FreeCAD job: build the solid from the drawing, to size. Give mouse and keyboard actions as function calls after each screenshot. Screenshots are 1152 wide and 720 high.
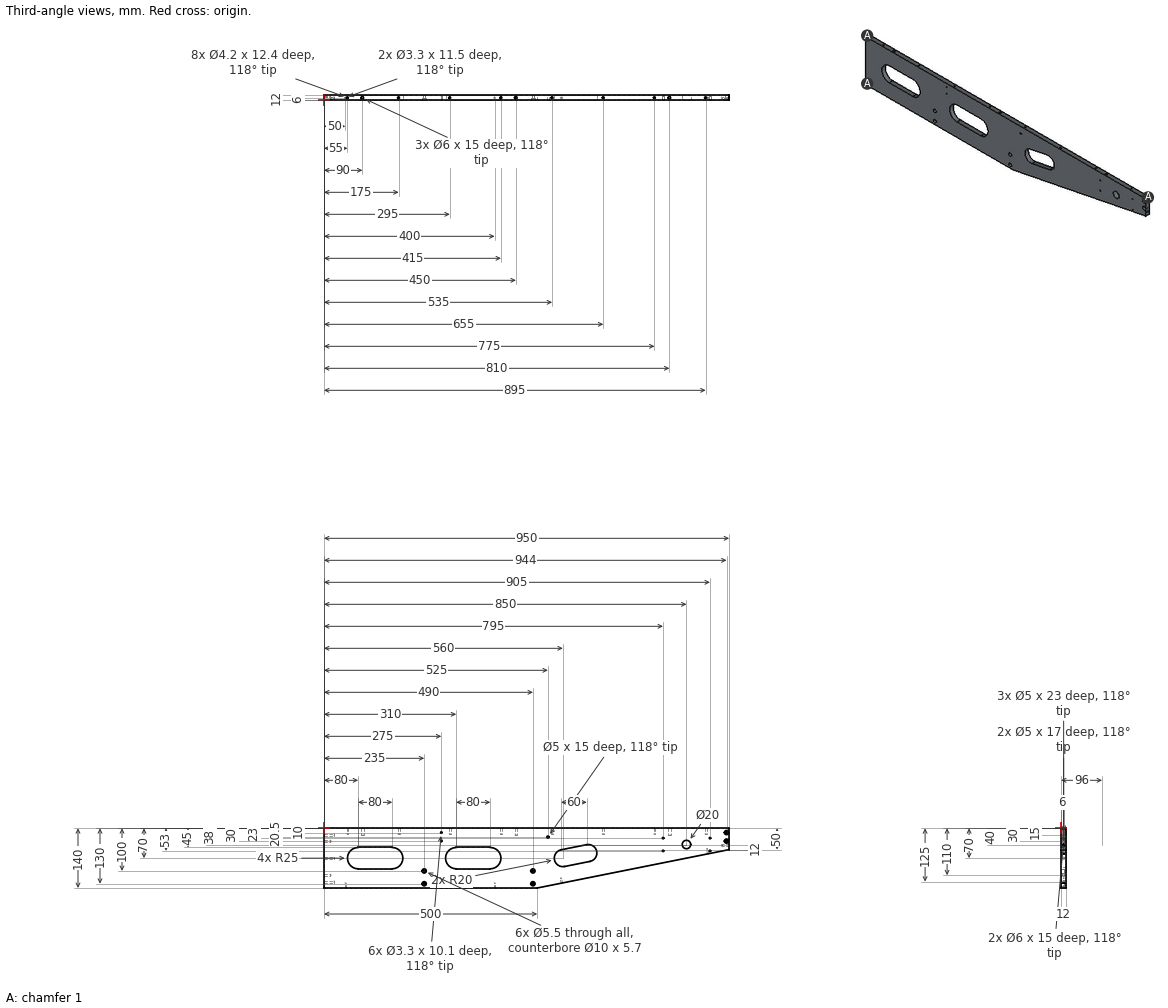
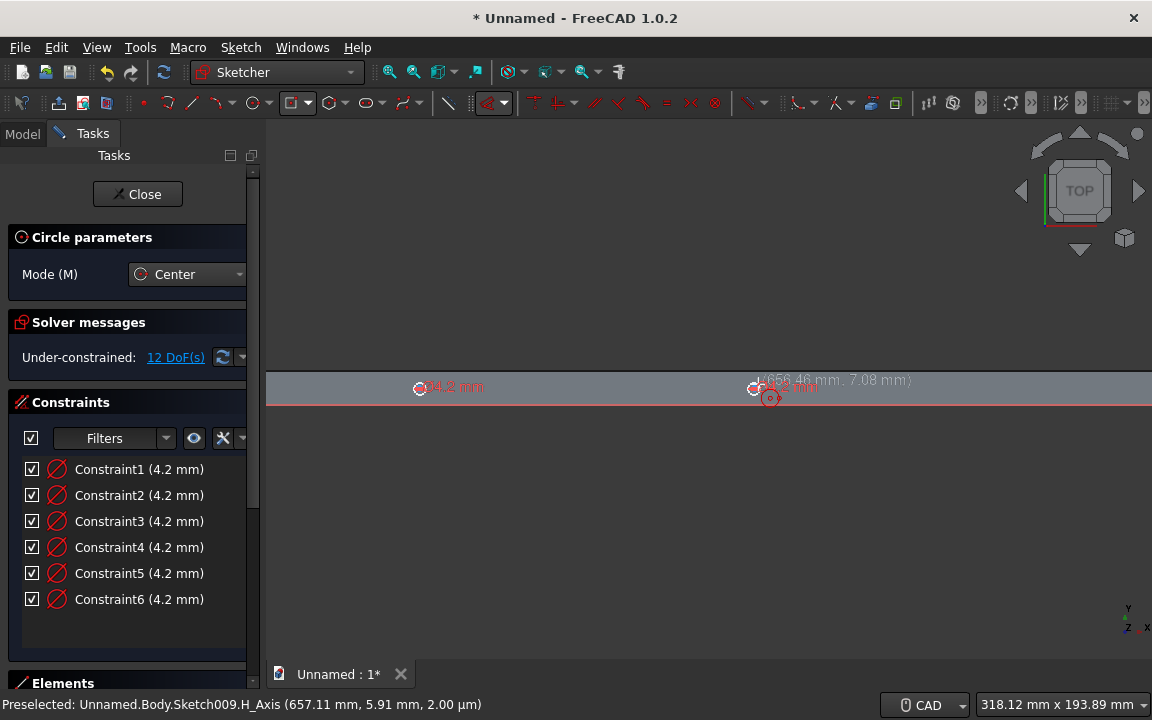
scroll(757, 388, down, 8)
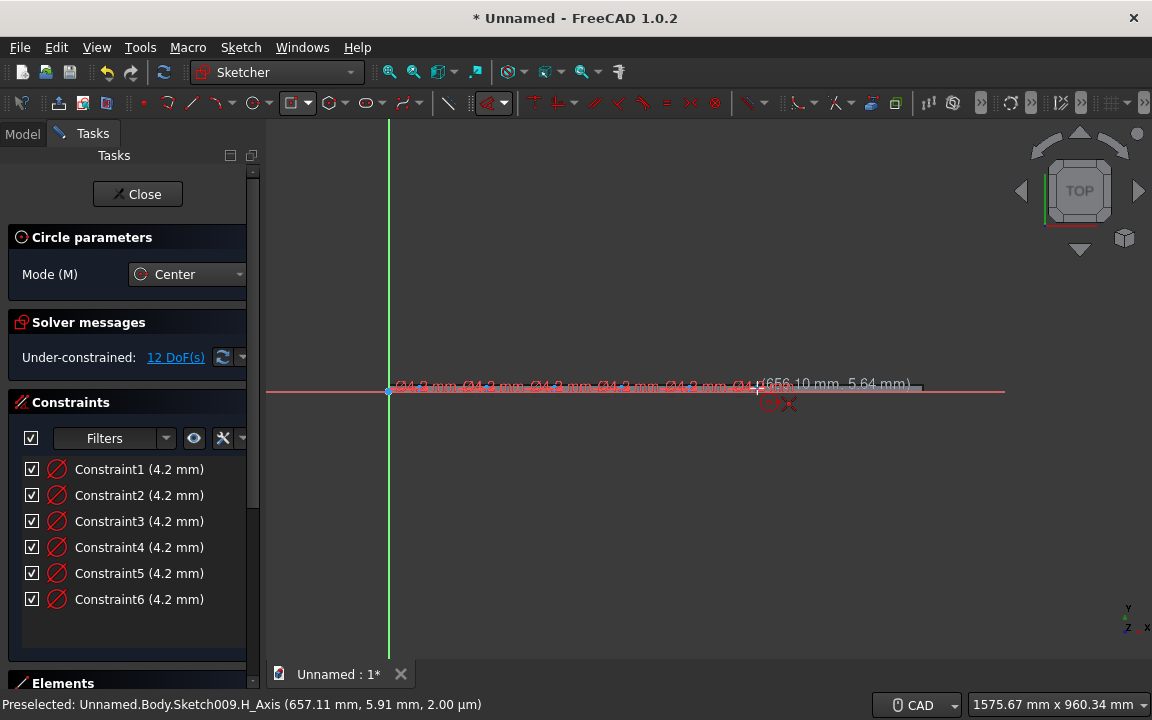
scroll(824, 388, up, 15)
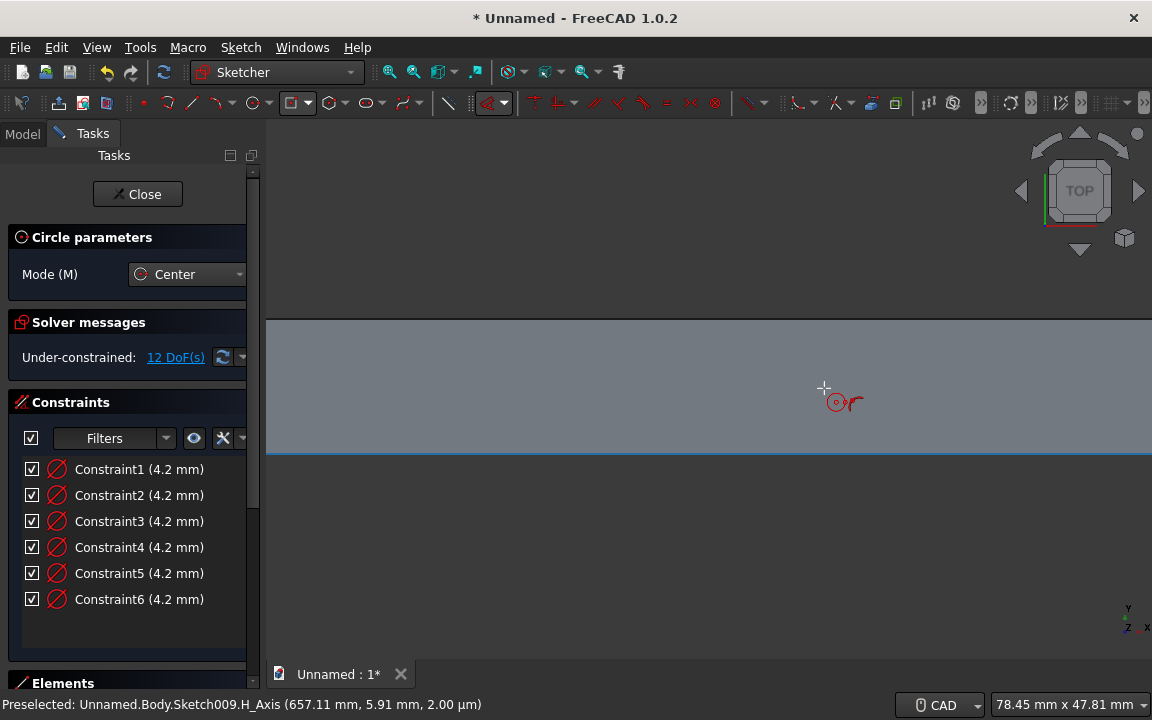
scroll(824, 388, down, 15)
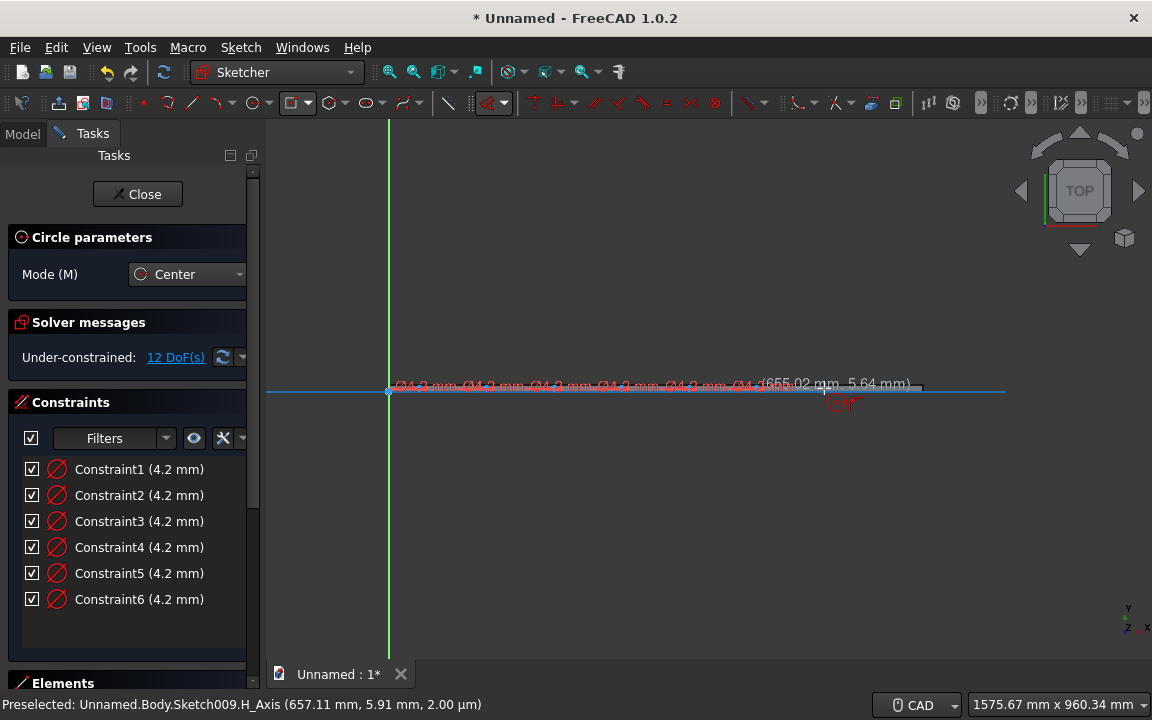
scroll(824, 388, up, 8)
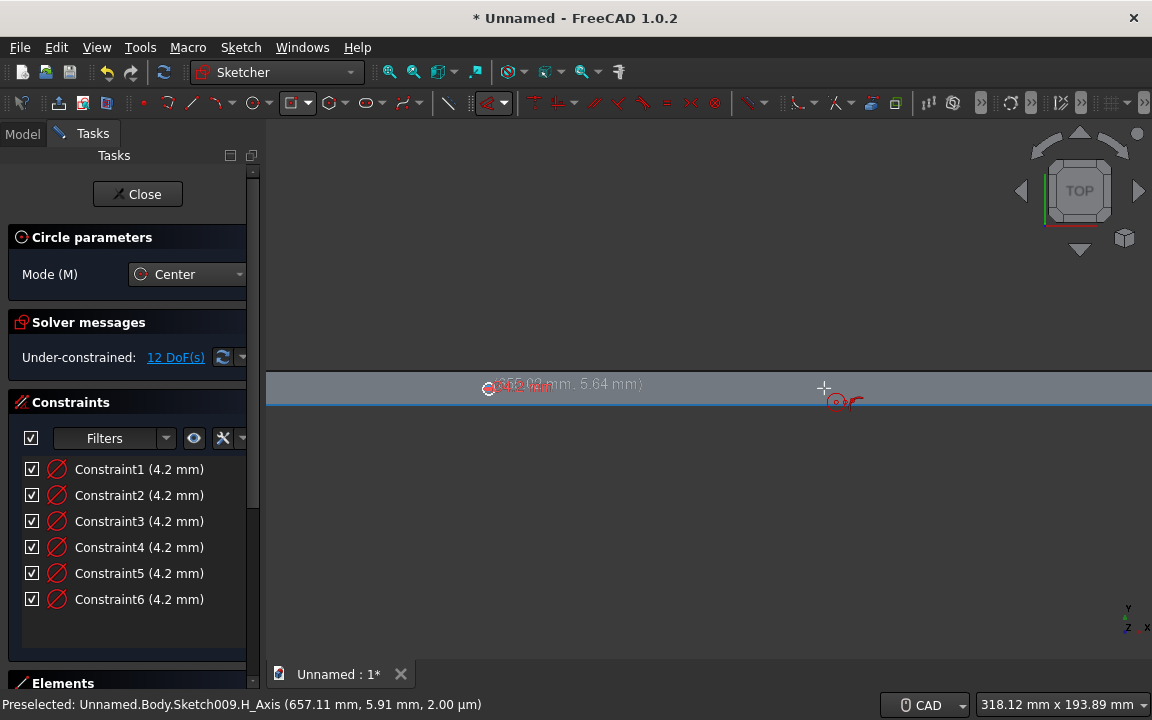
click(823, 388)
move(827, 384)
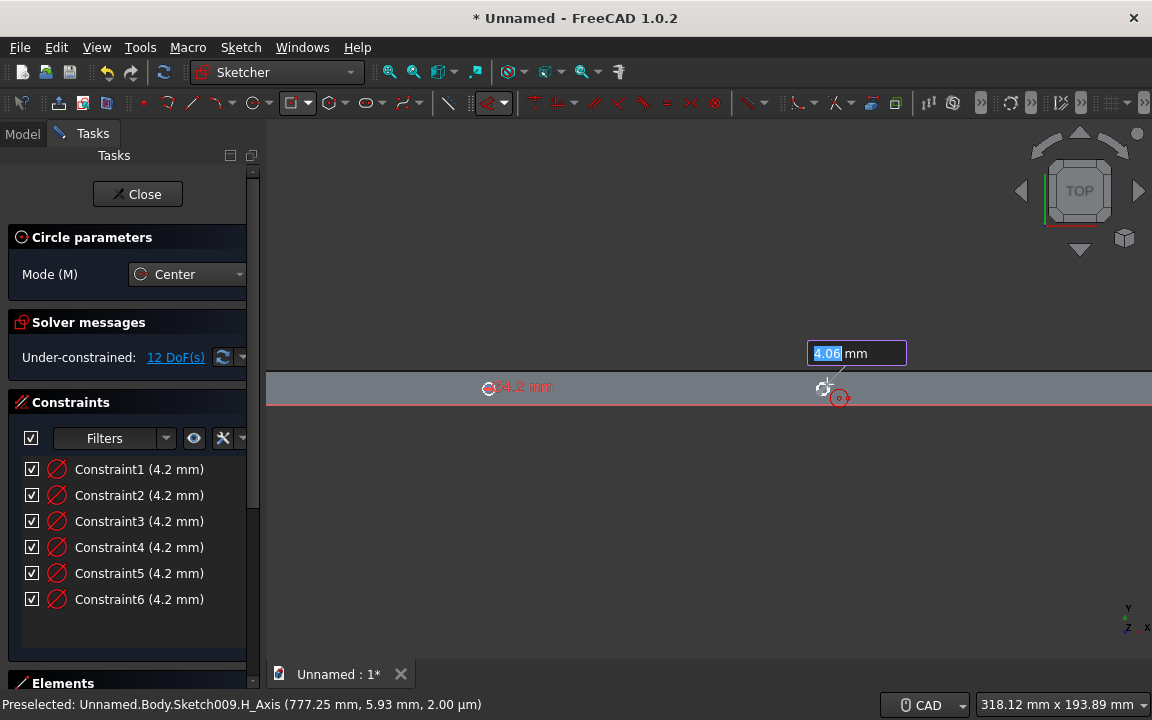
text(4.2)
key(Return)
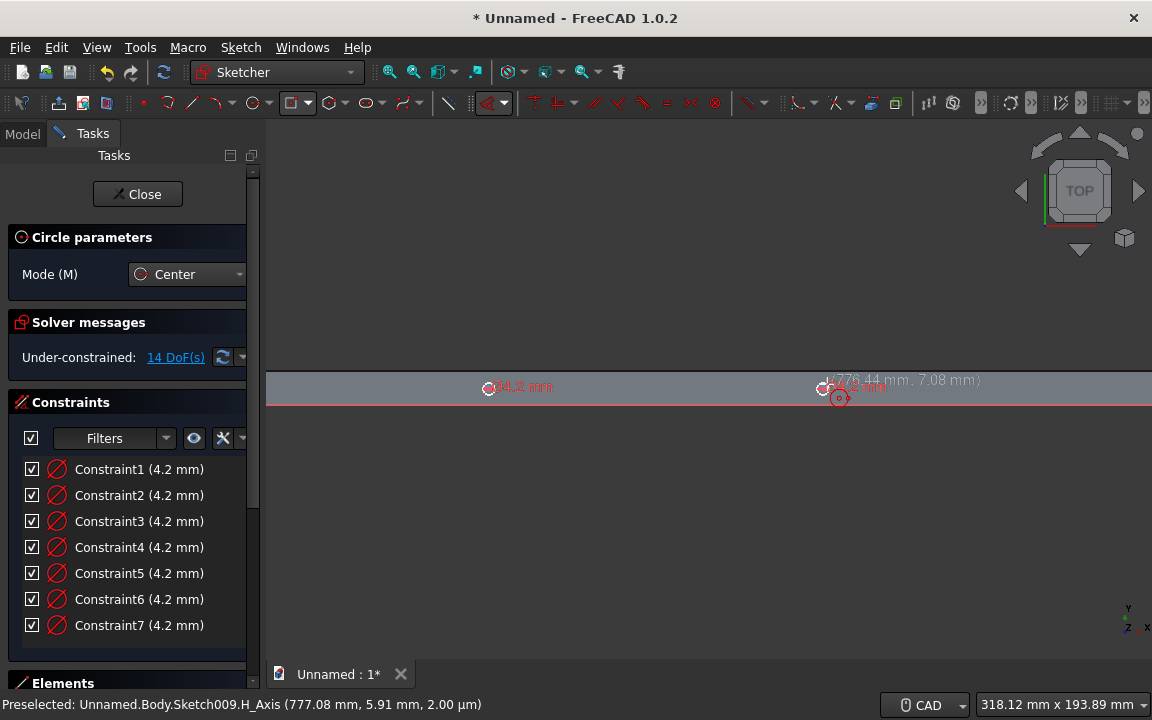
scroll(824, 388, down, 8)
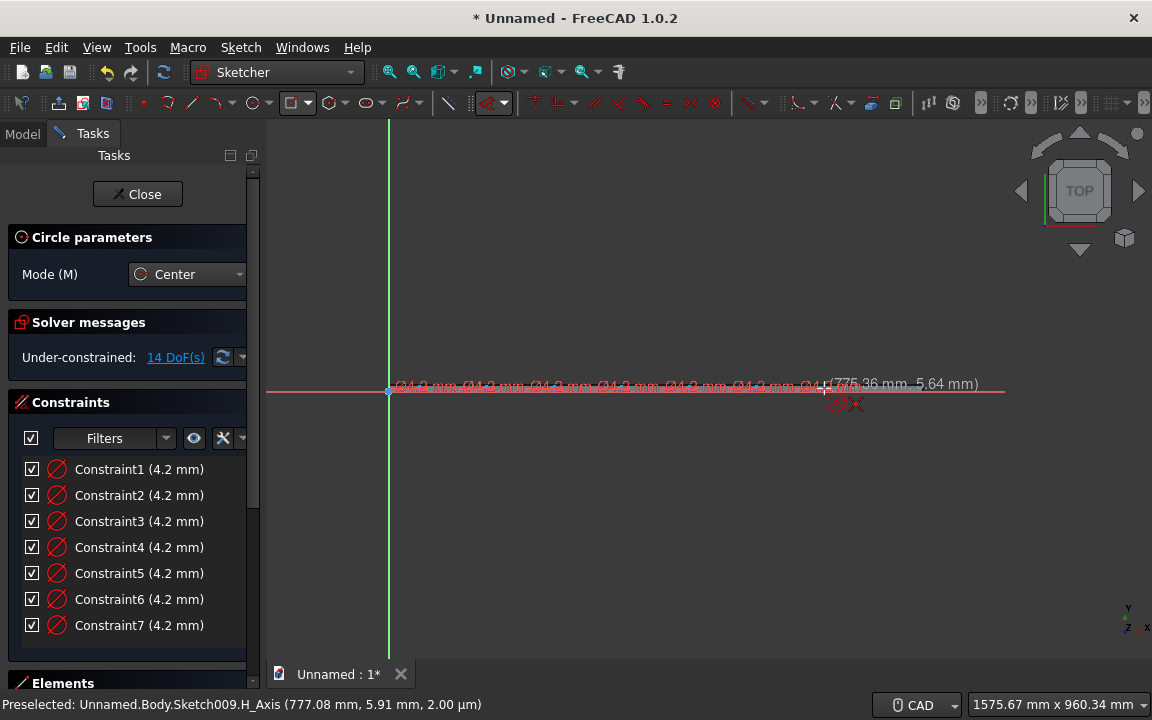
scroll(892, 388, up, 15)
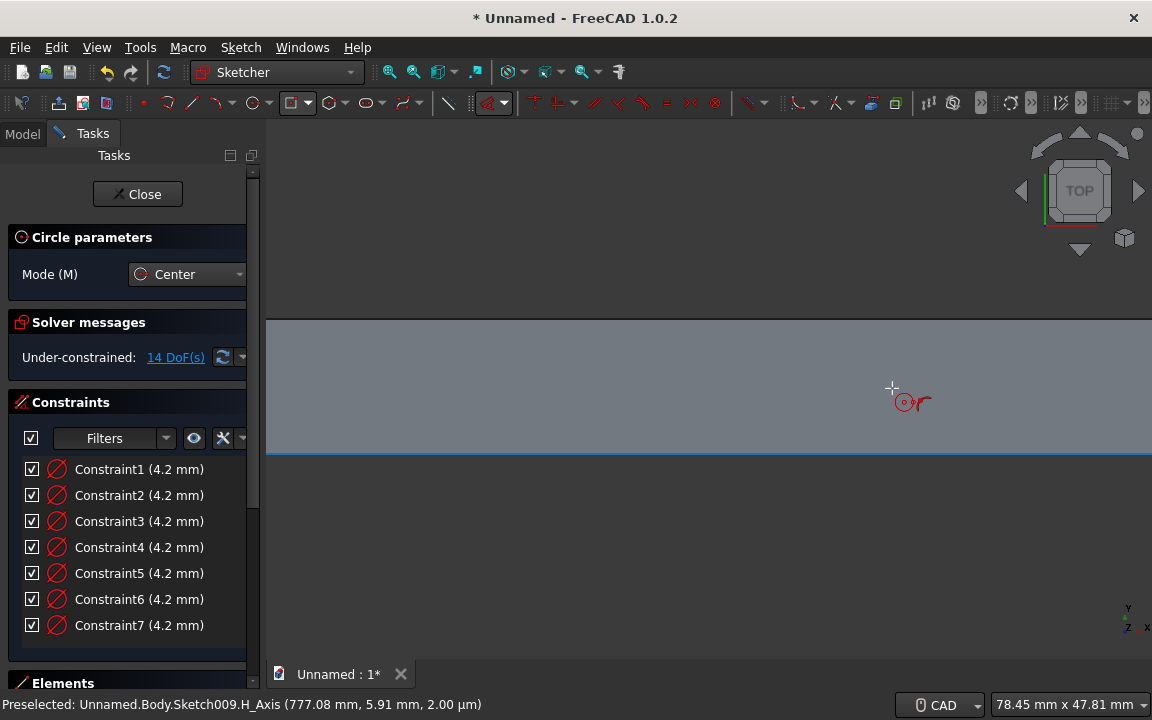
scroll(892, 388, down, 15)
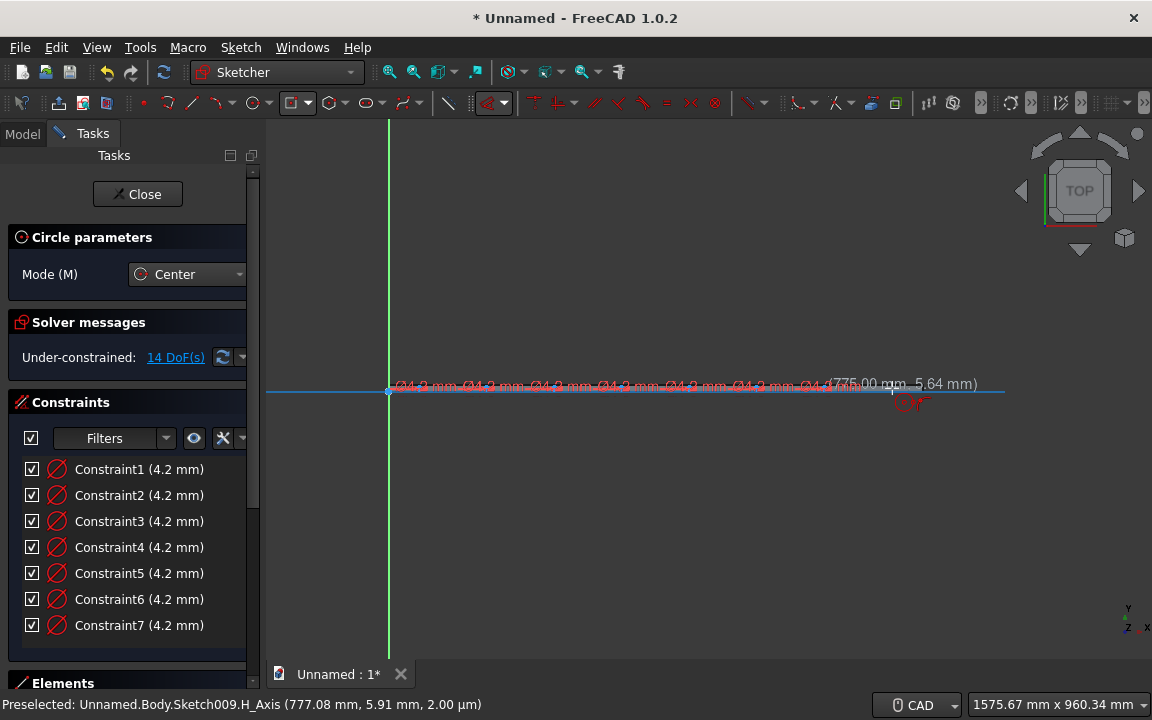
scroll(892, 388, up, 8)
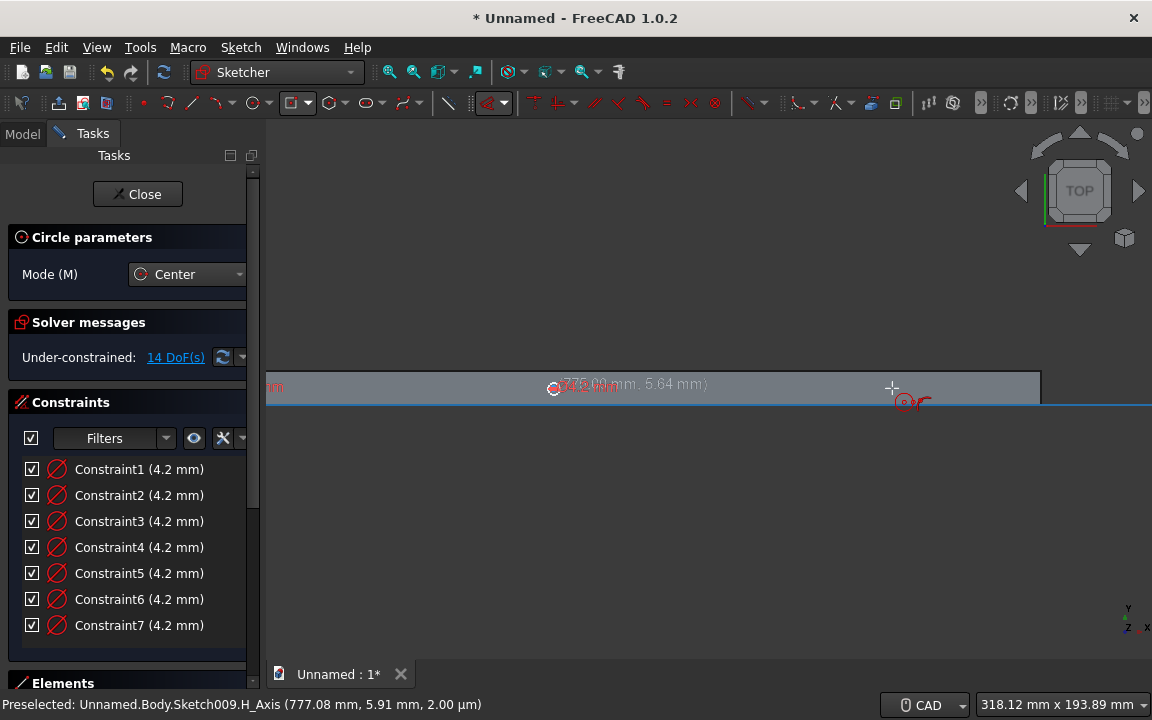
click(888, 388)
move(892, 384)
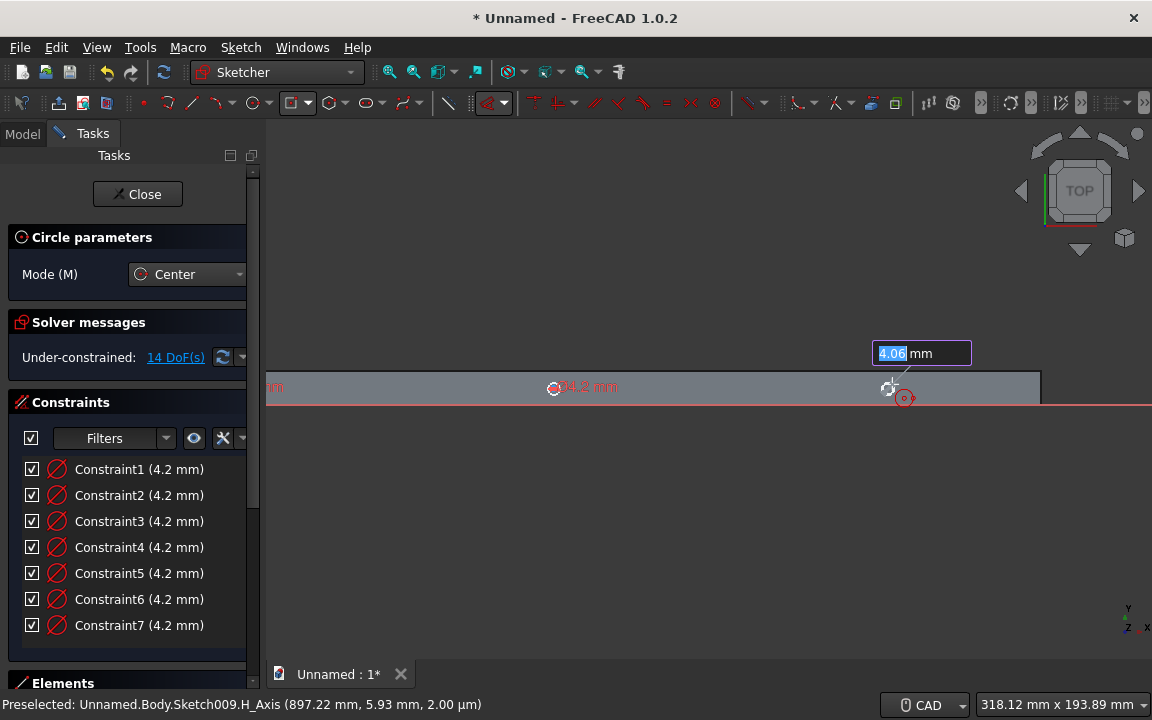
text(4.2)
key(Return)
key(Escape)